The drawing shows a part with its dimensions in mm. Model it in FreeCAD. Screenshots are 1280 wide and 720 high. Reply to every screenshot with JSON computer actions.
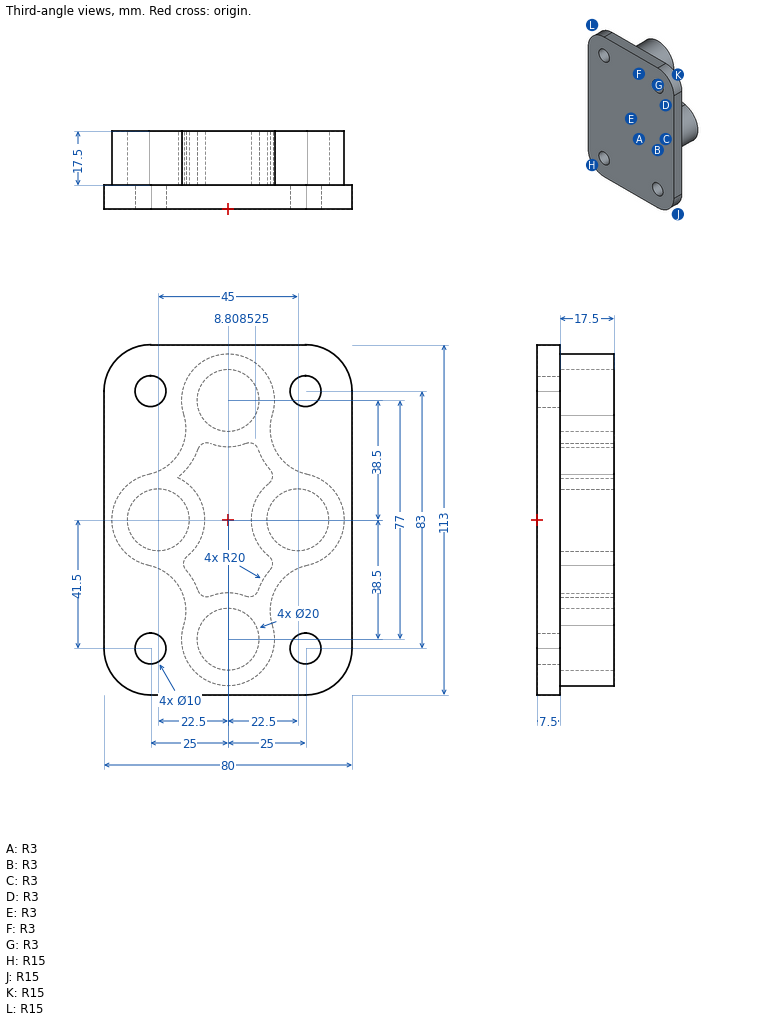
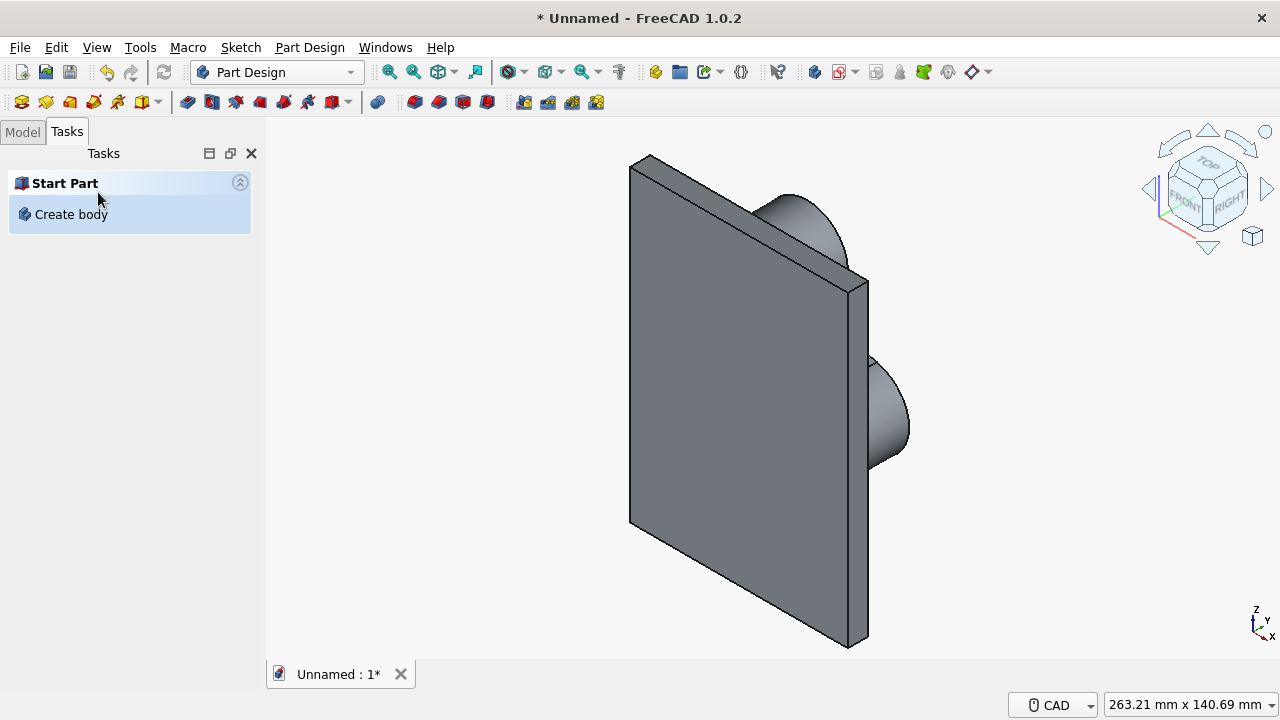
{"action": "key", "text": "1"}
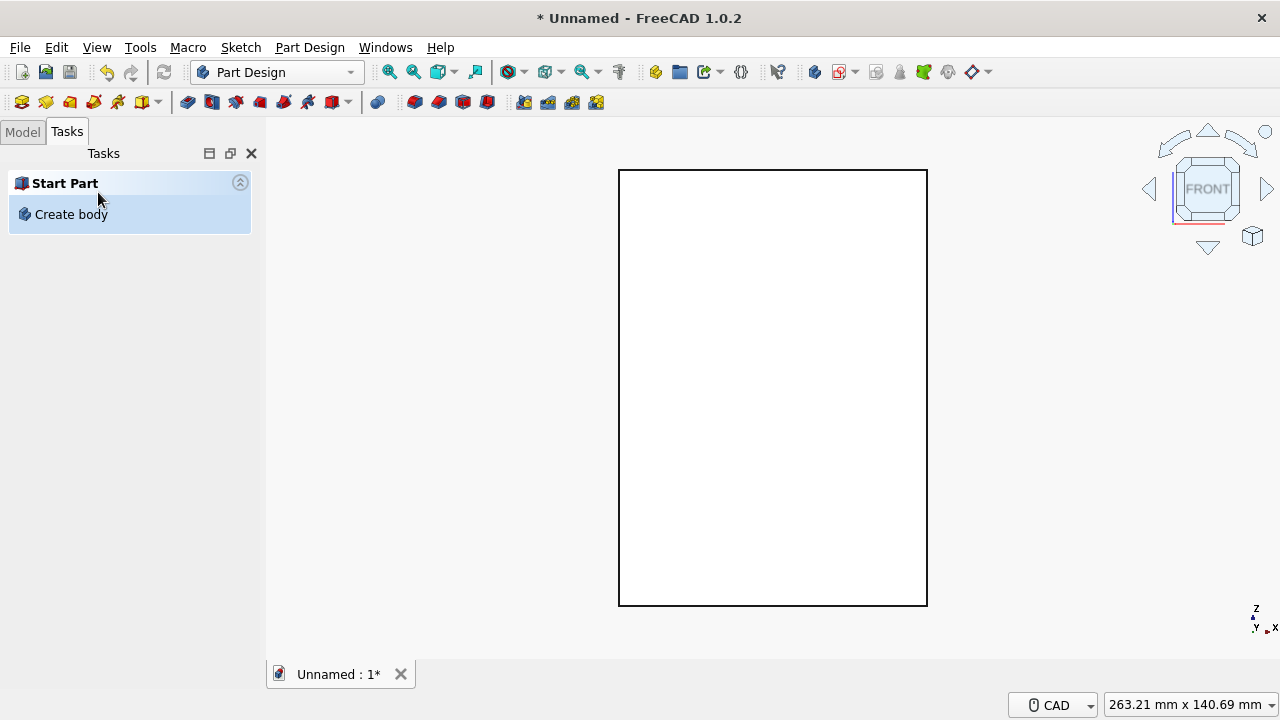
{"action": "key", "text": "3"}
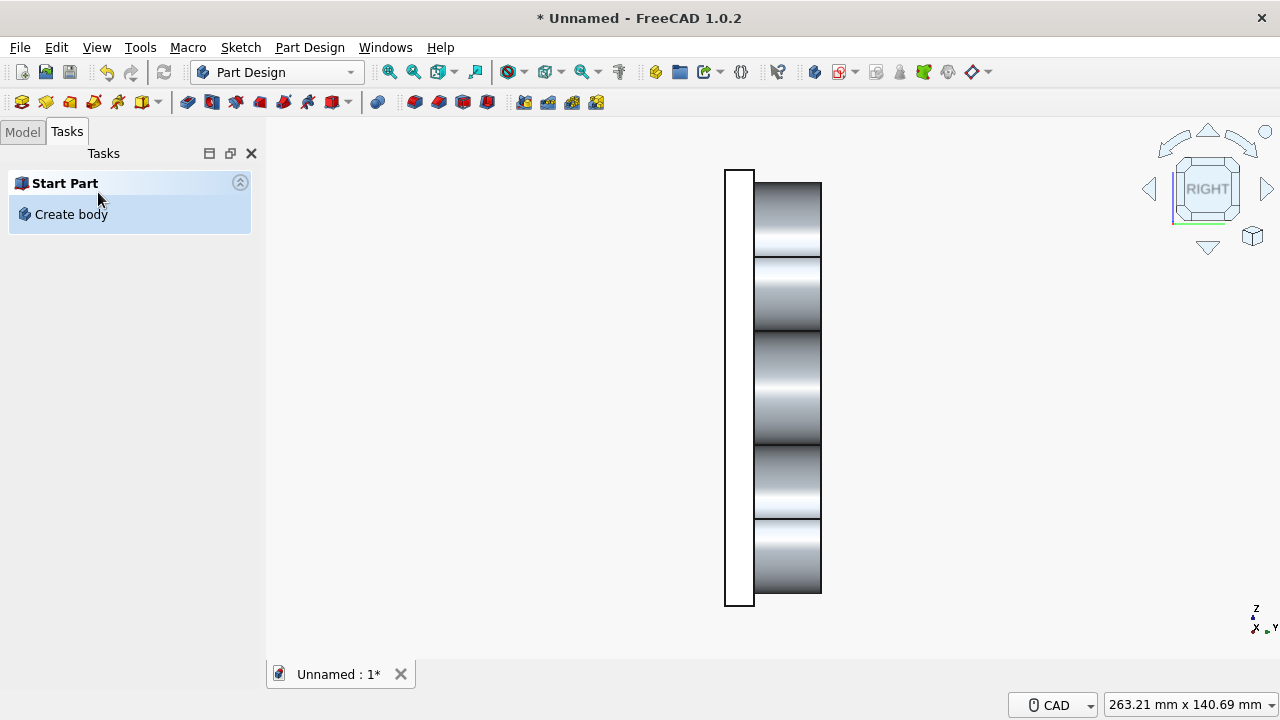
{"action": "key", "text": "5"}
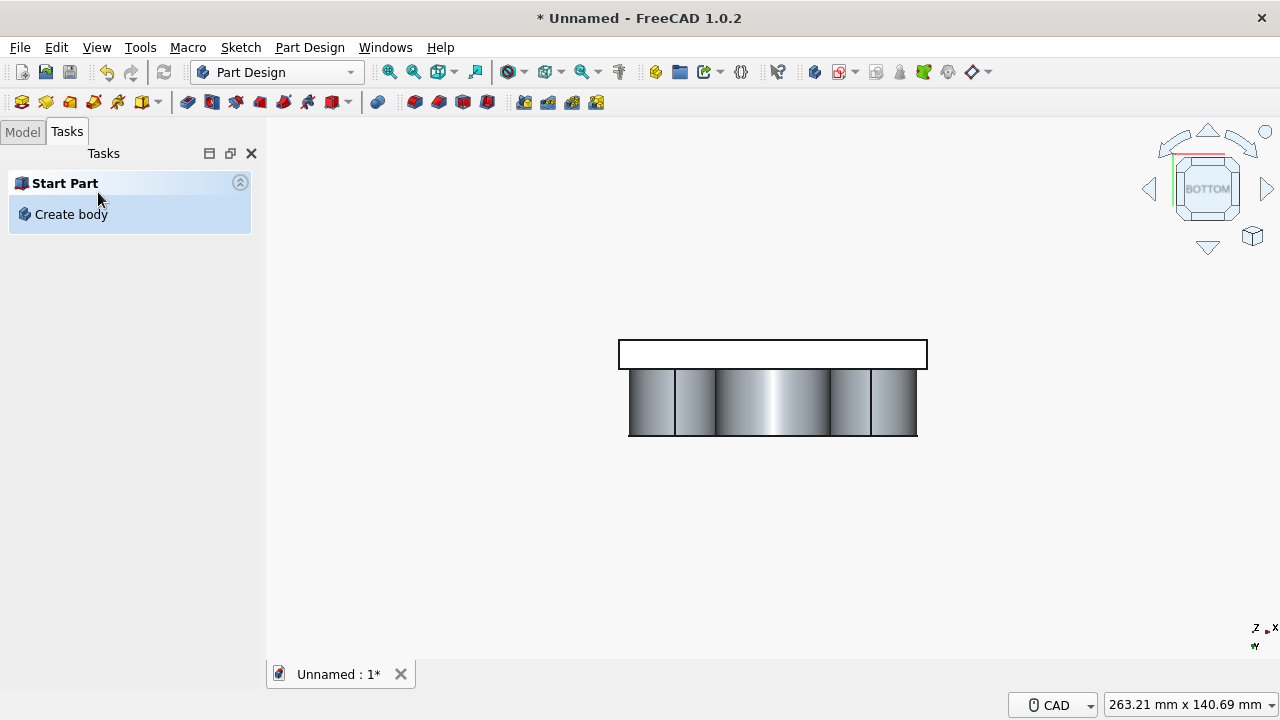
{"action": "key", "text": "v f"}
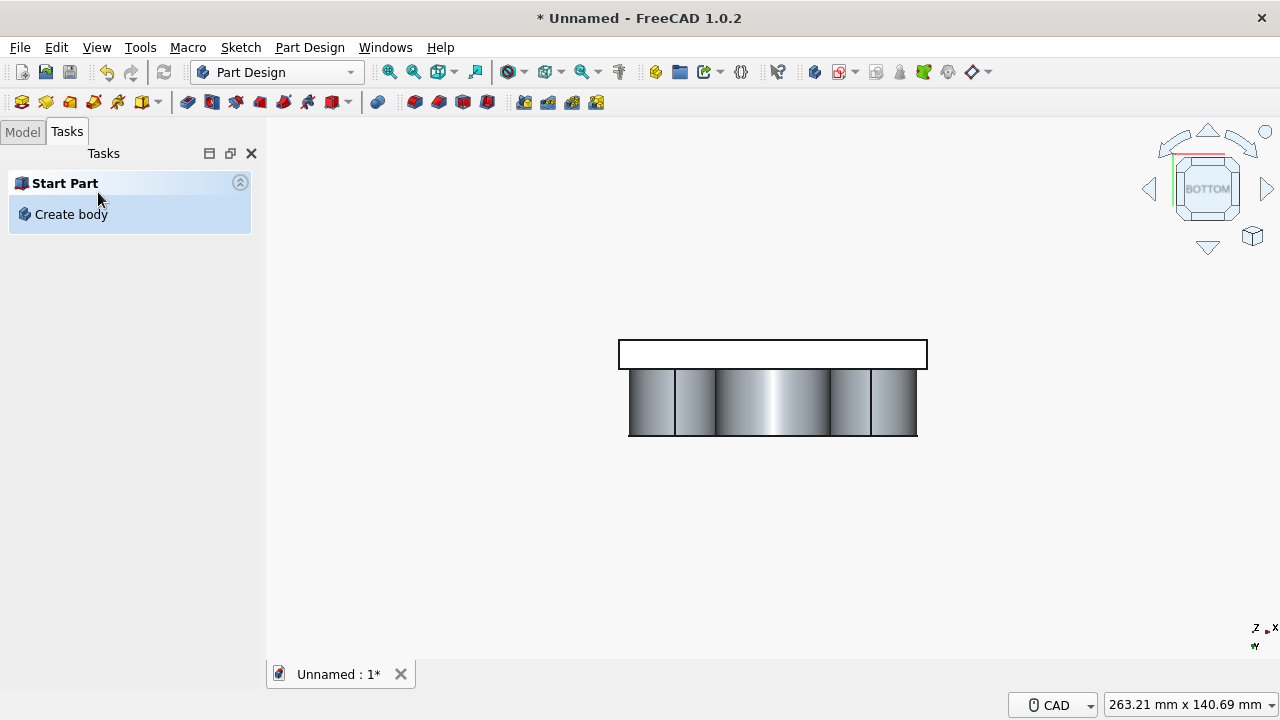
{"action": "key", "text": "4"}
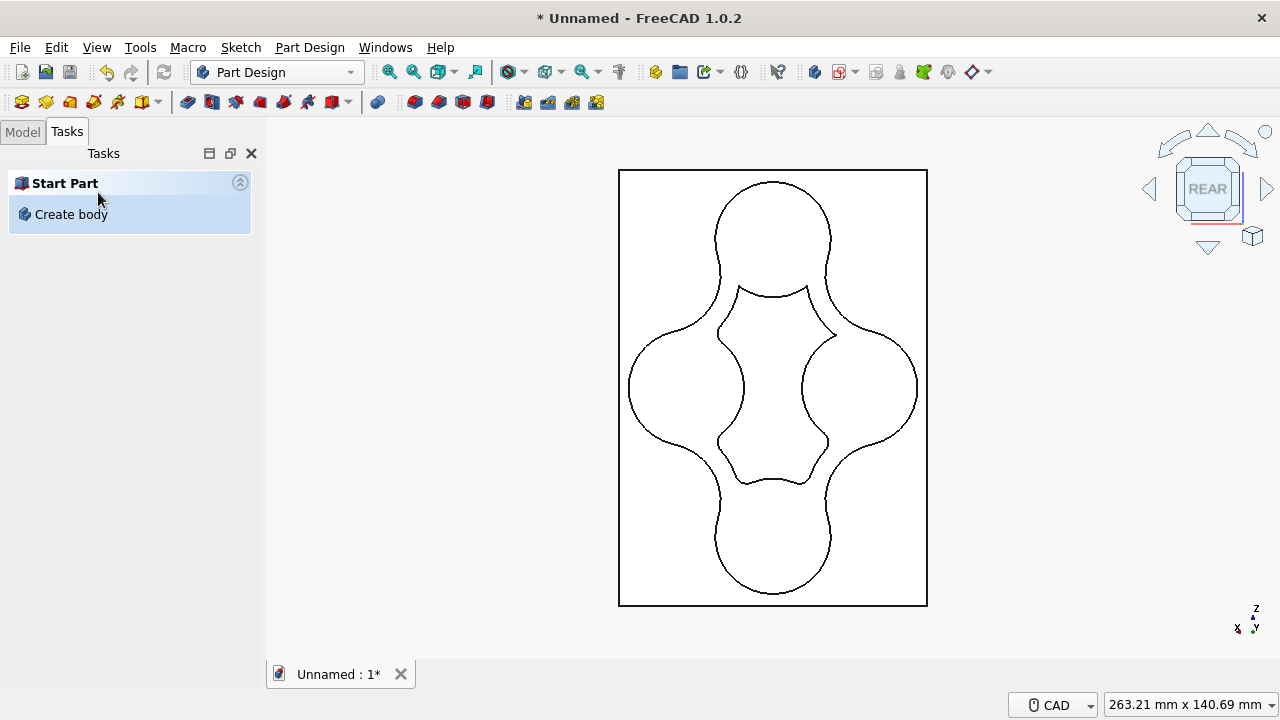
{"action": "key", "text": "6"}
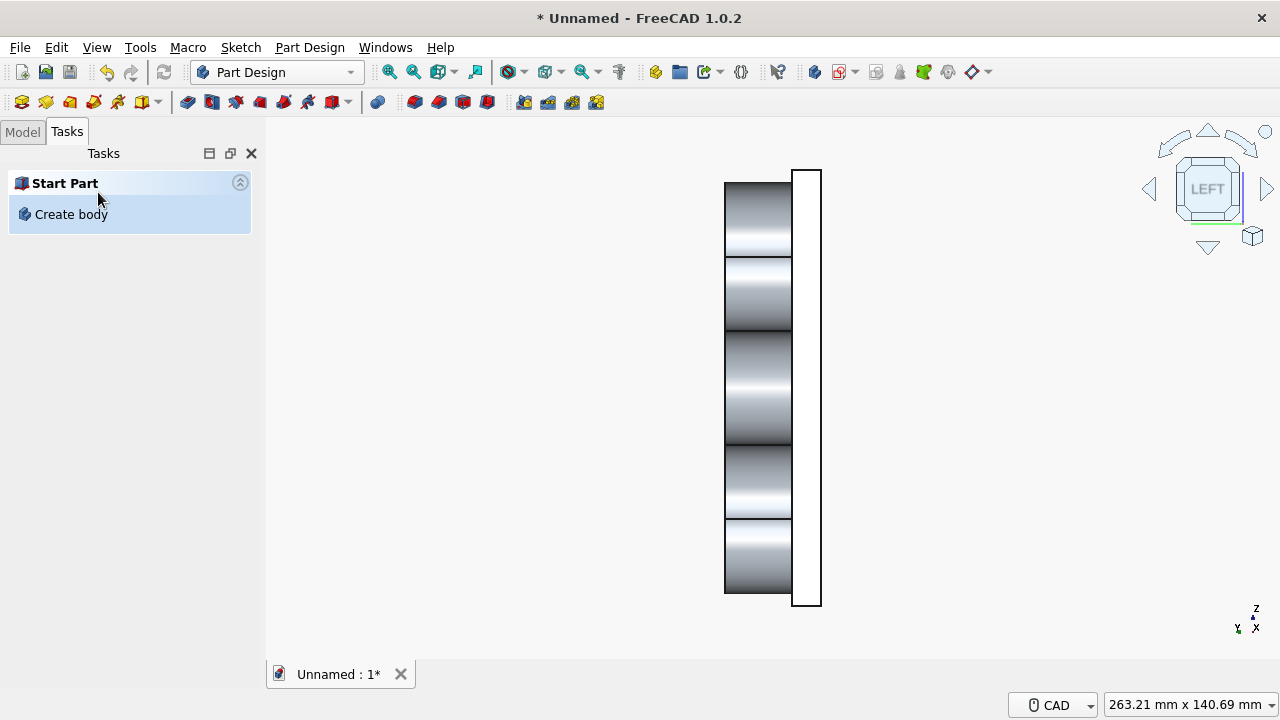
{"action": "key", "text": "v 3"}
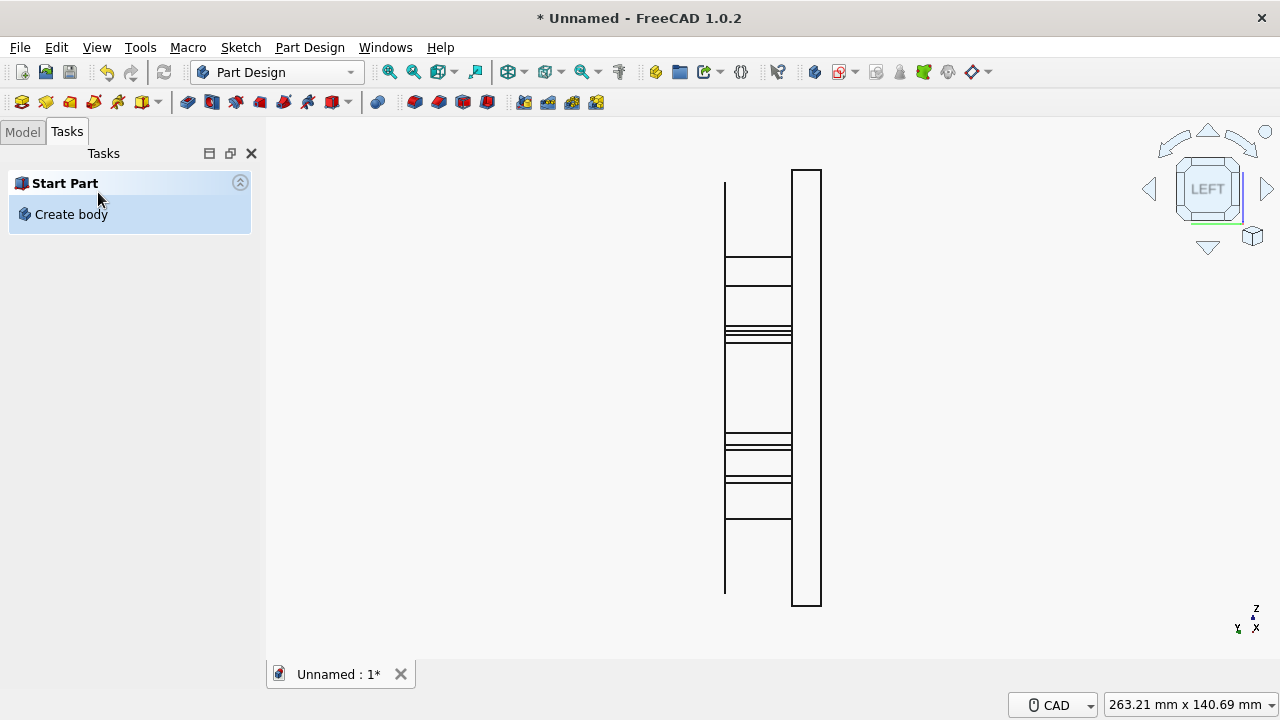
{"action": "key", "text": "0"}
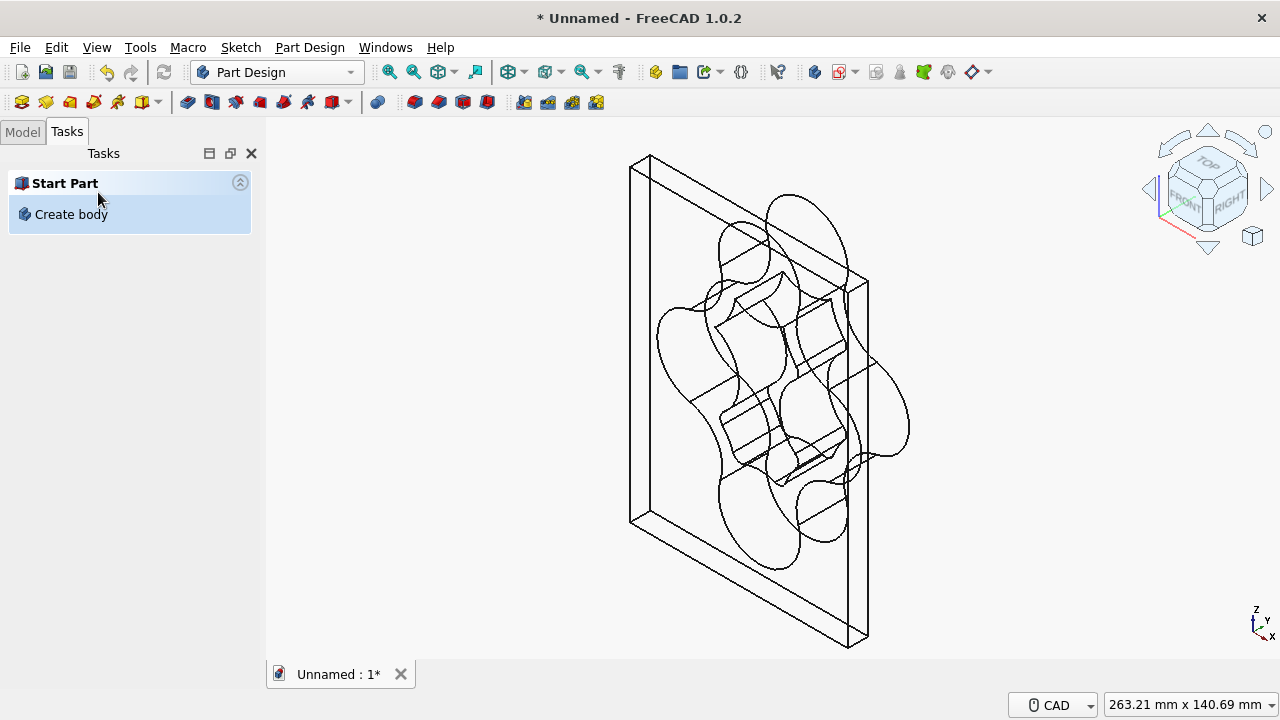
{"action": "left_click", "coordinate": [759, 284]}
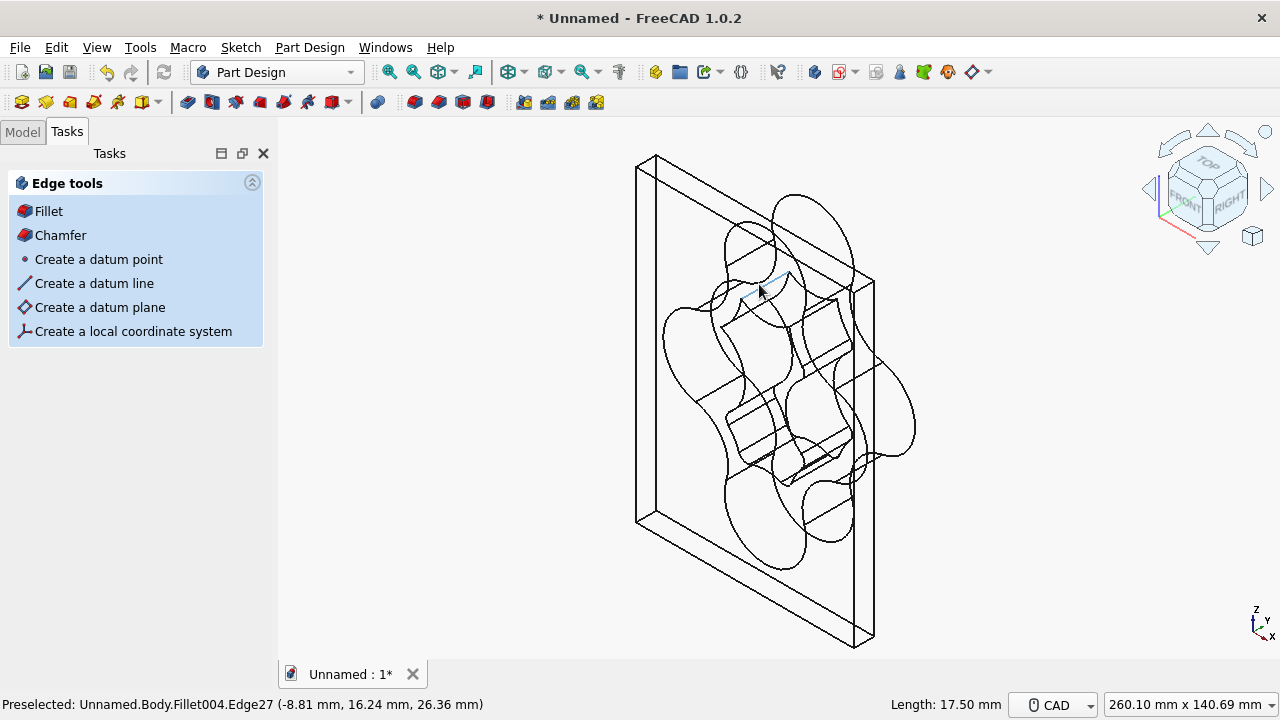
{"action": "key", "text": "v 1"}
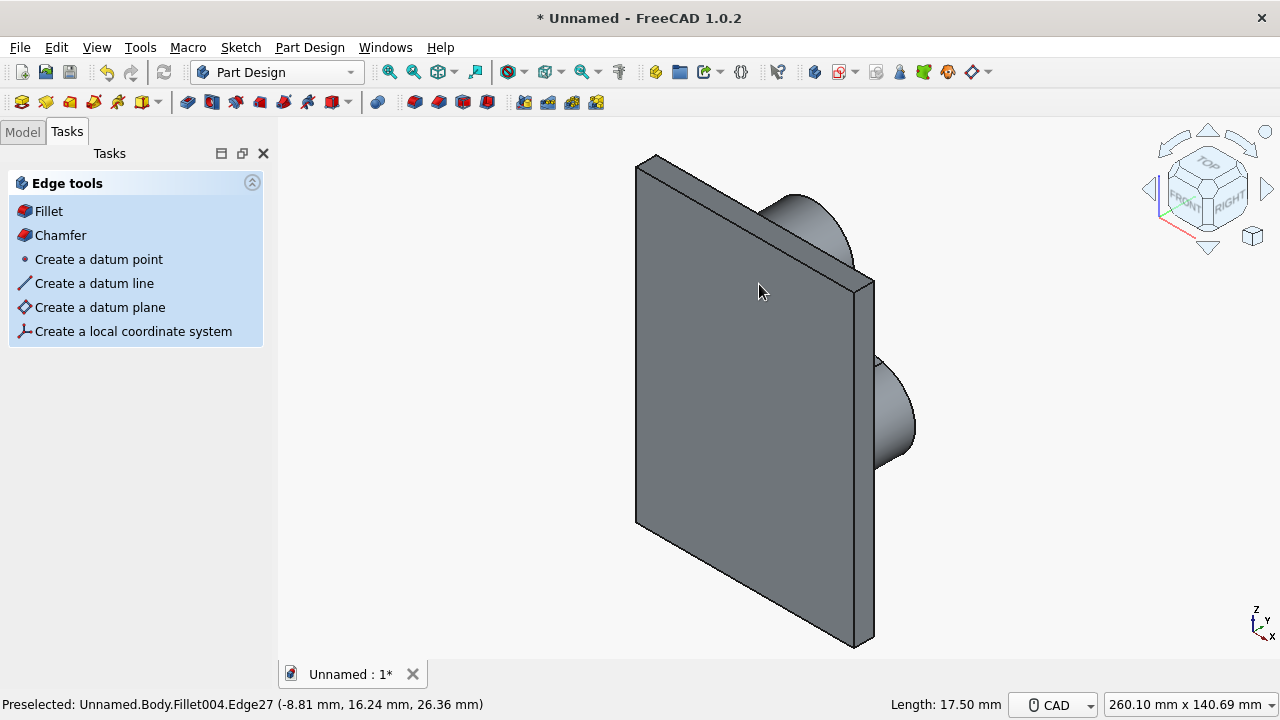
{"action": "left_click", "coordinate": [416, 102]}